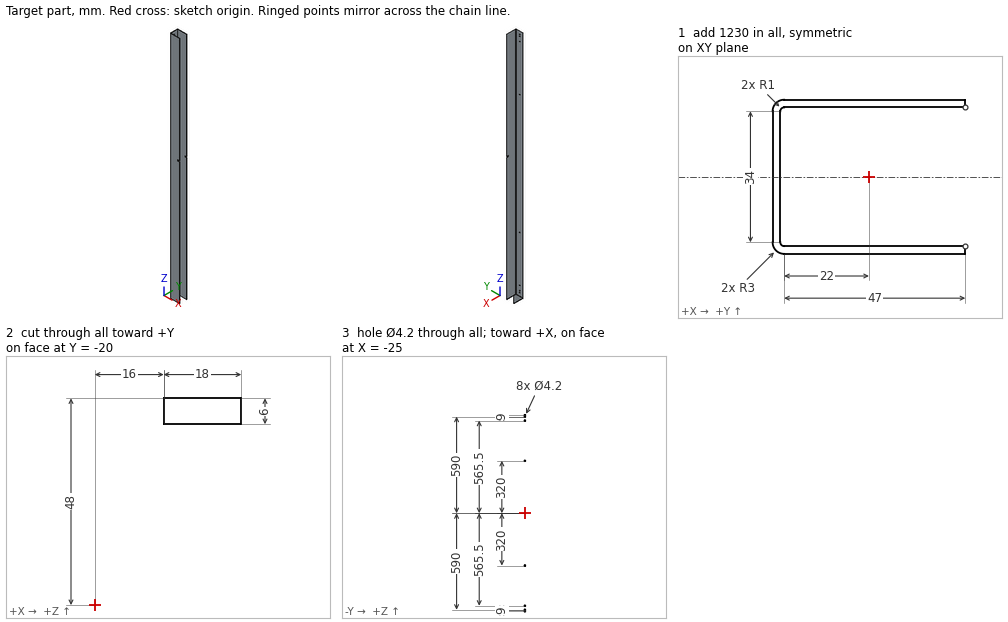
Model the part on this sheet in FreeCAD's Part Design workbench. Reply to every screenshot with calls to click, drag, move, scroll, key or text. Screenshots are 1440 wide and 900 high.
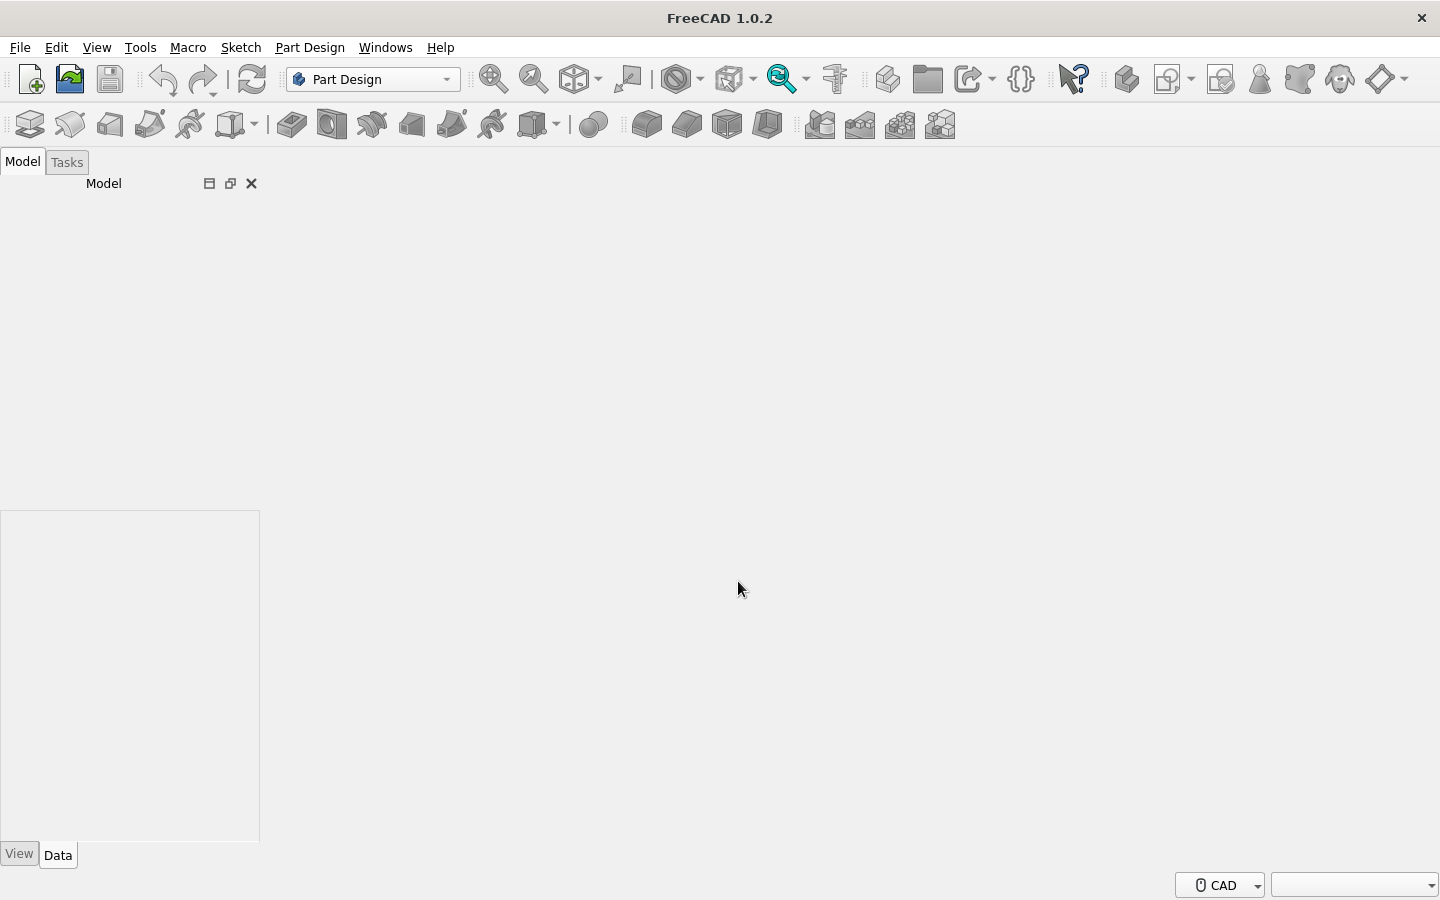
key(ctrl+n)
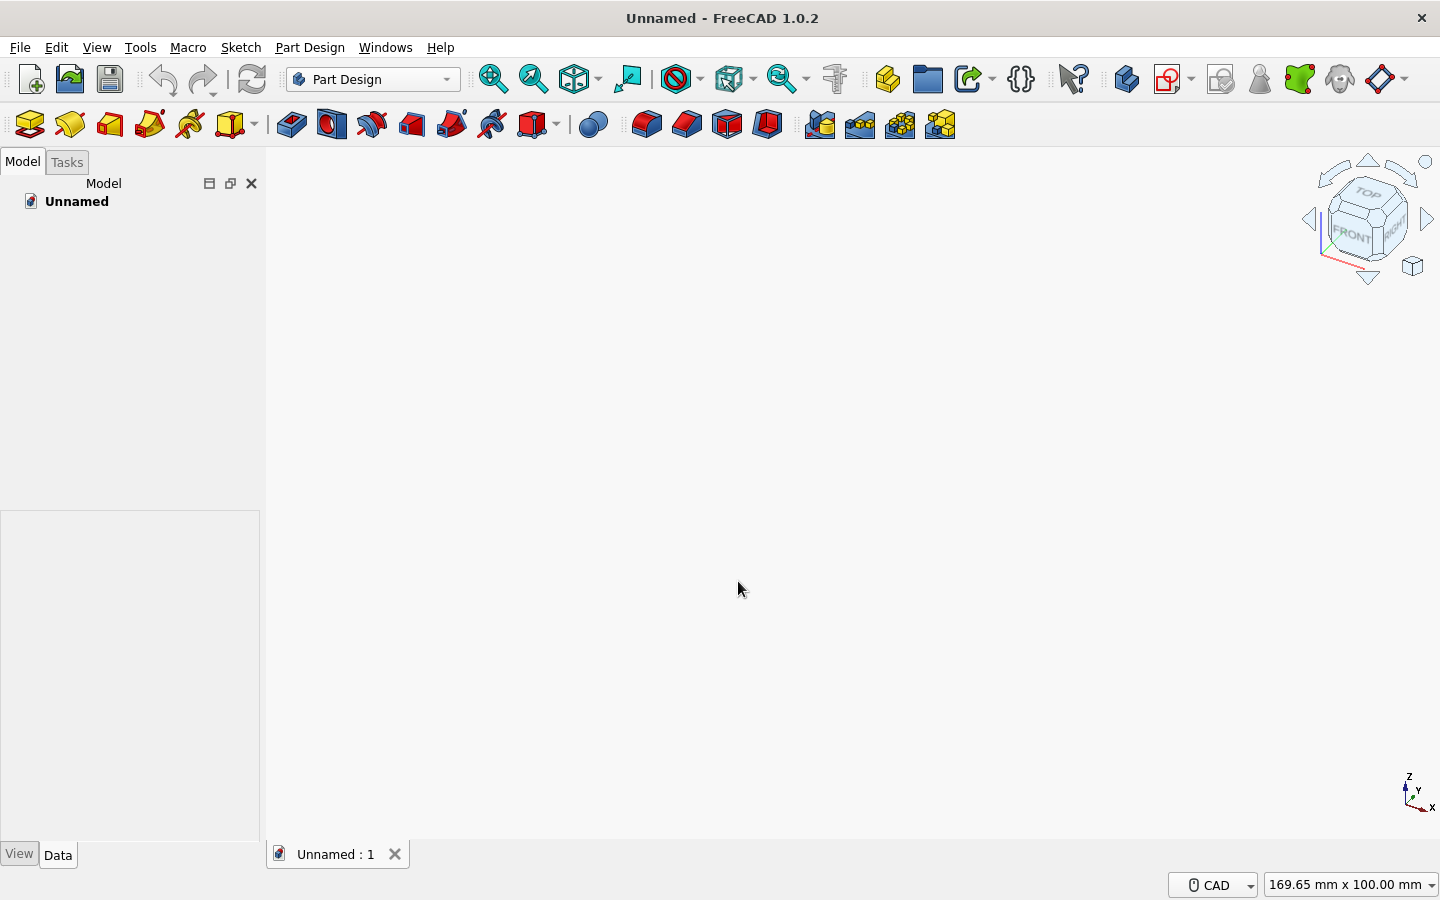
click(1168, 80)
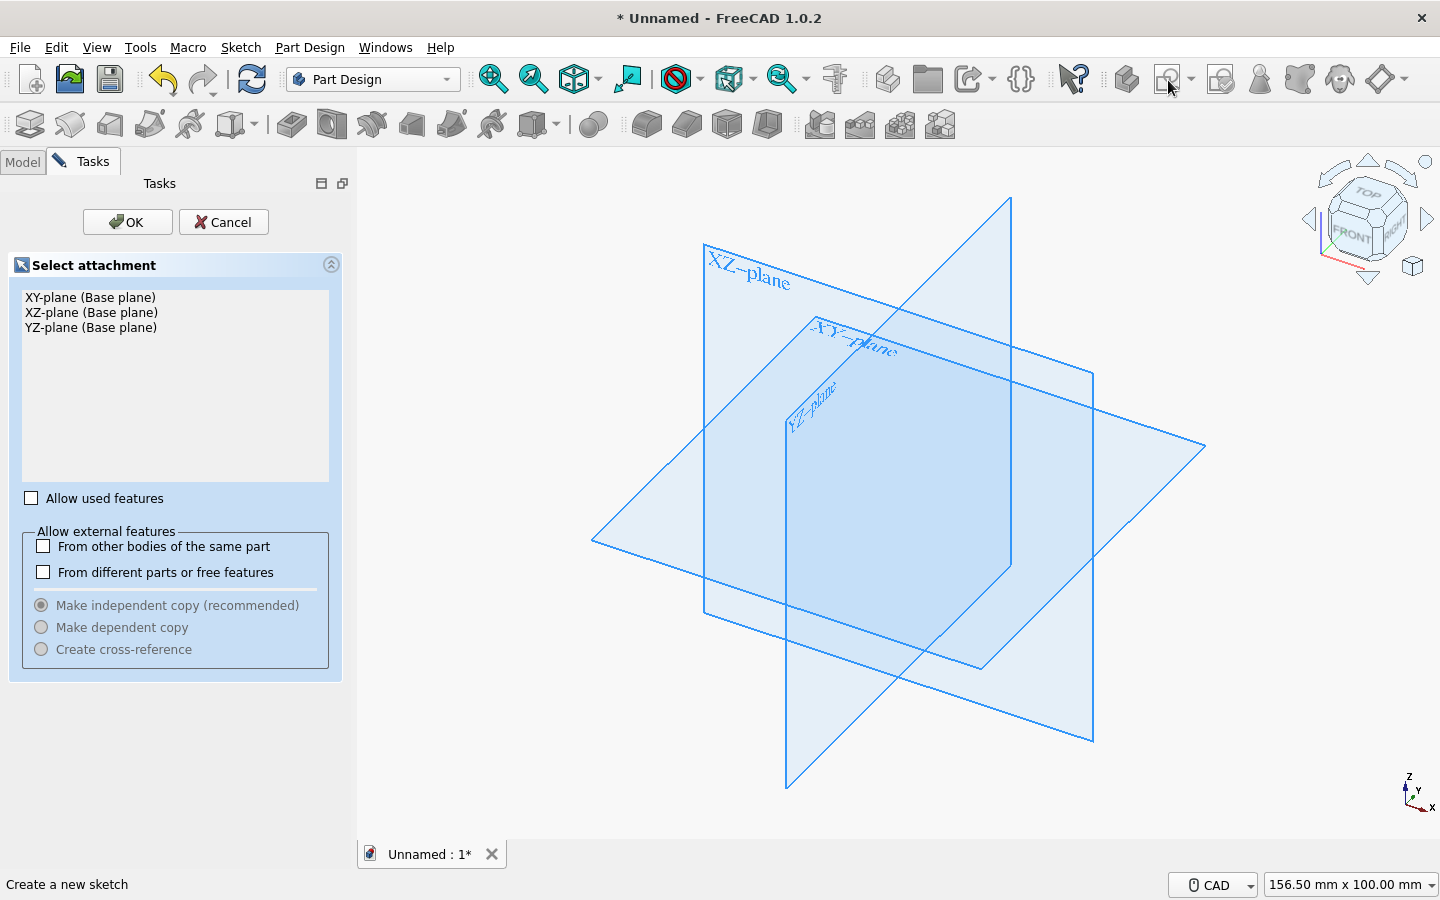
click(82, 298)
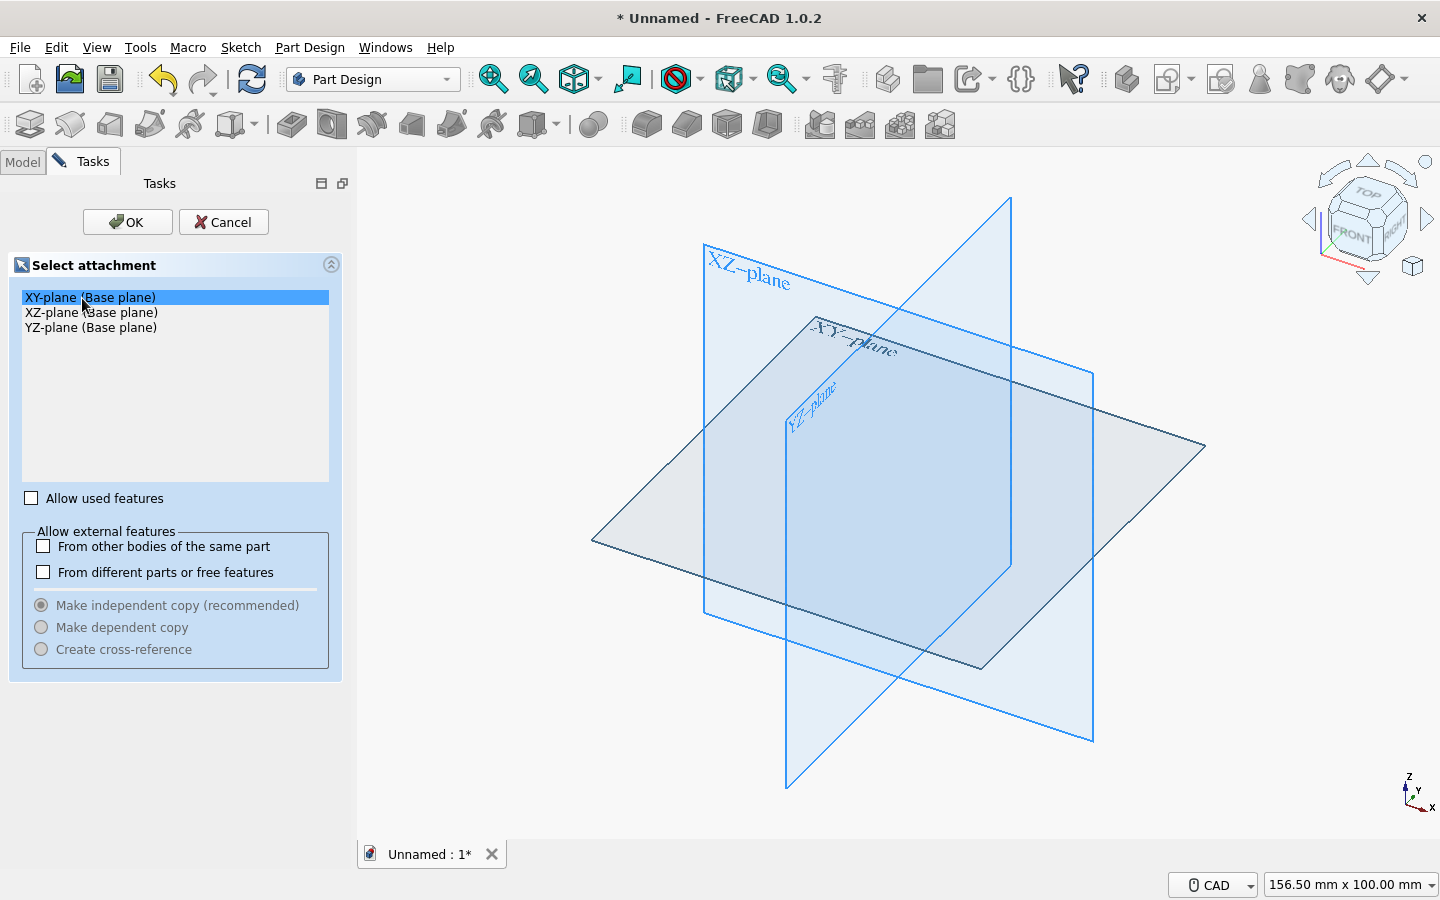
click(128, 222)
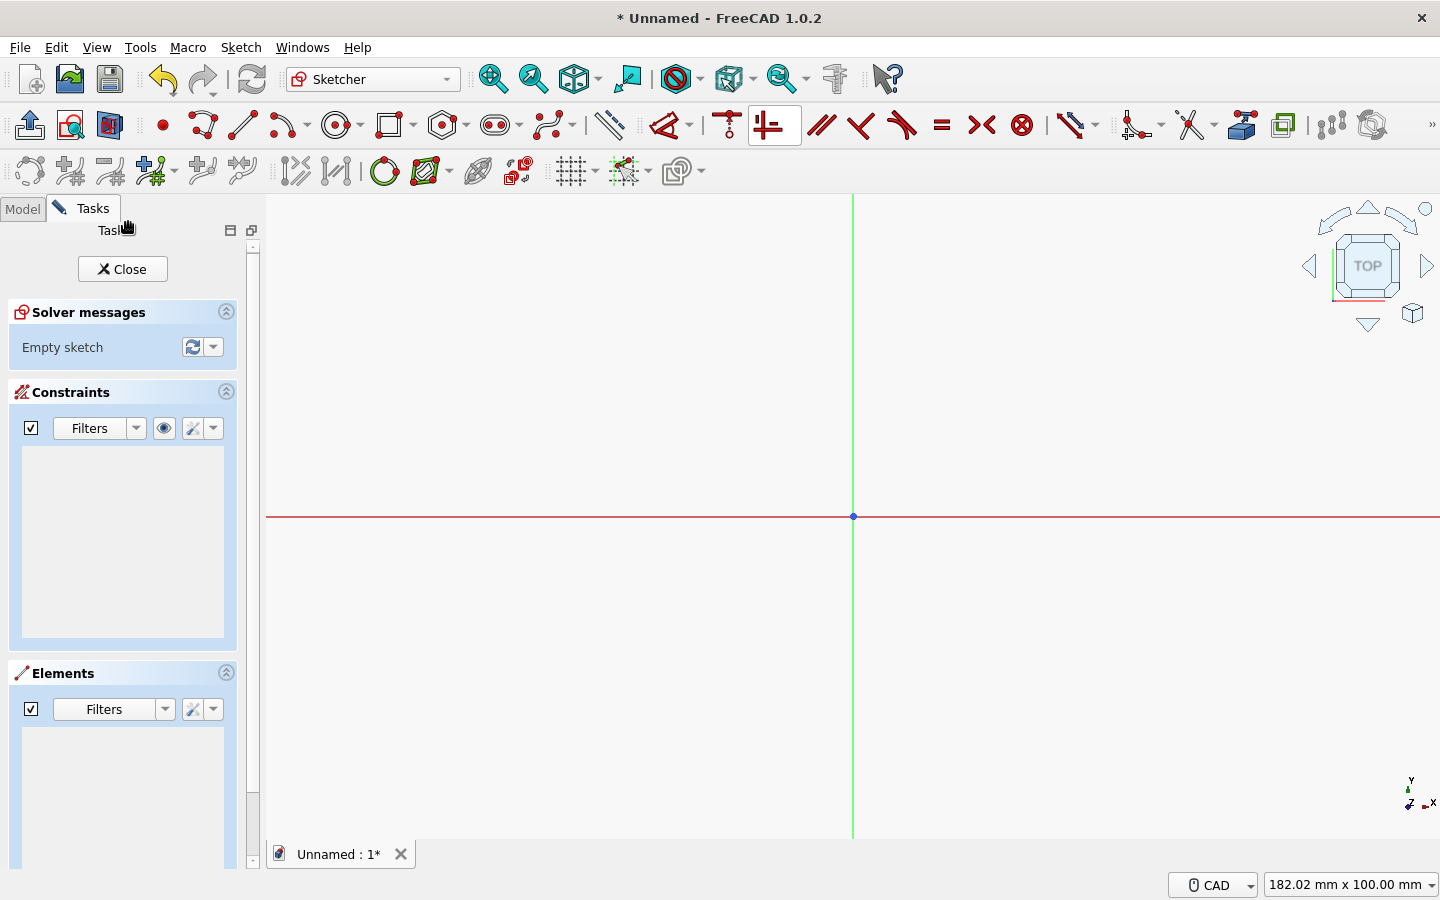
scroll(992, 517, up, 2)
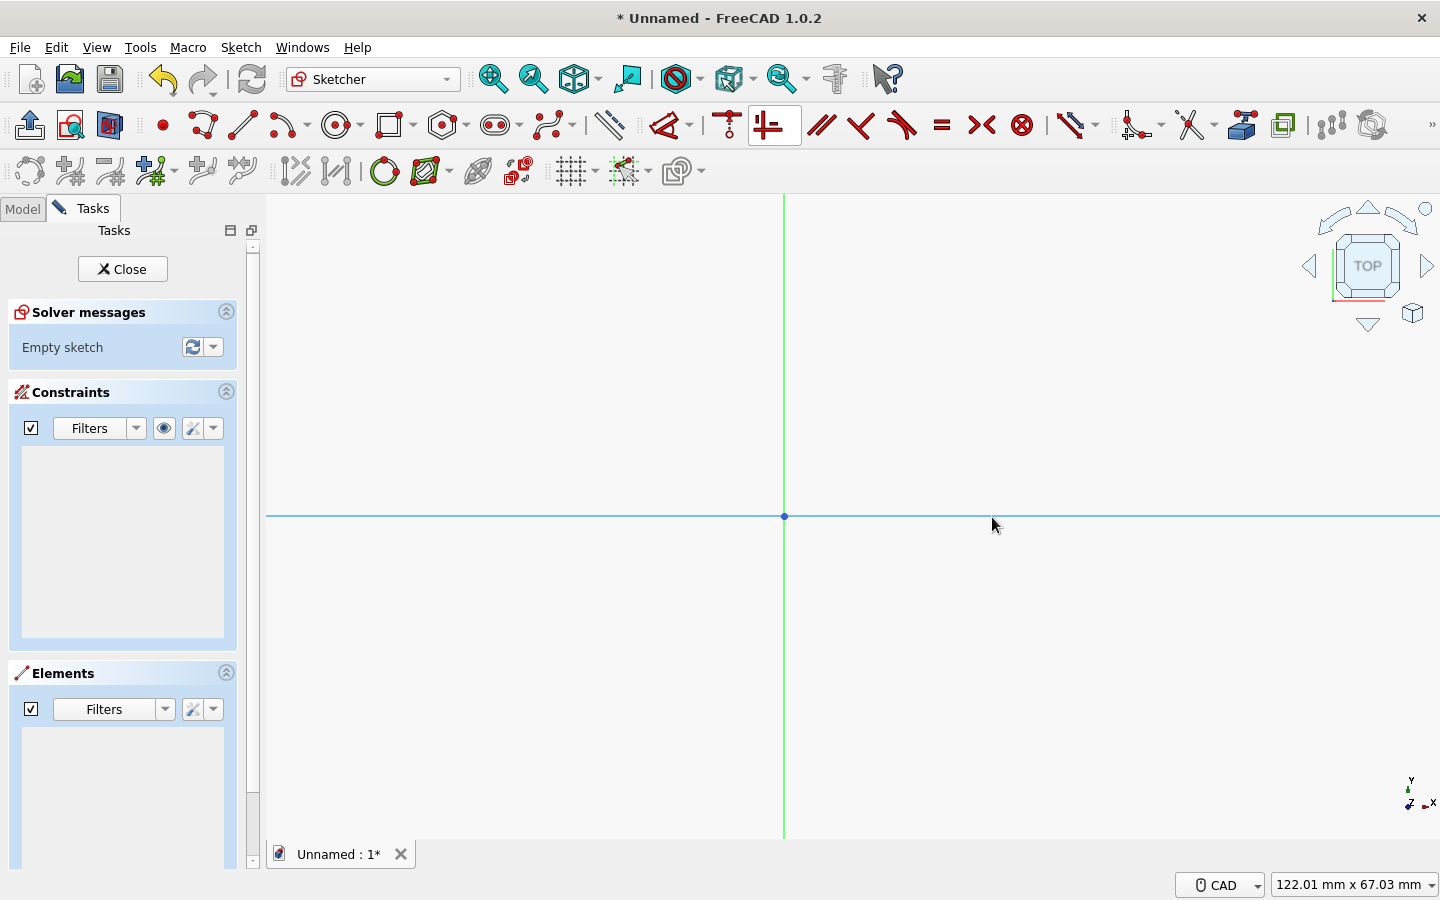
key(g)
key(m)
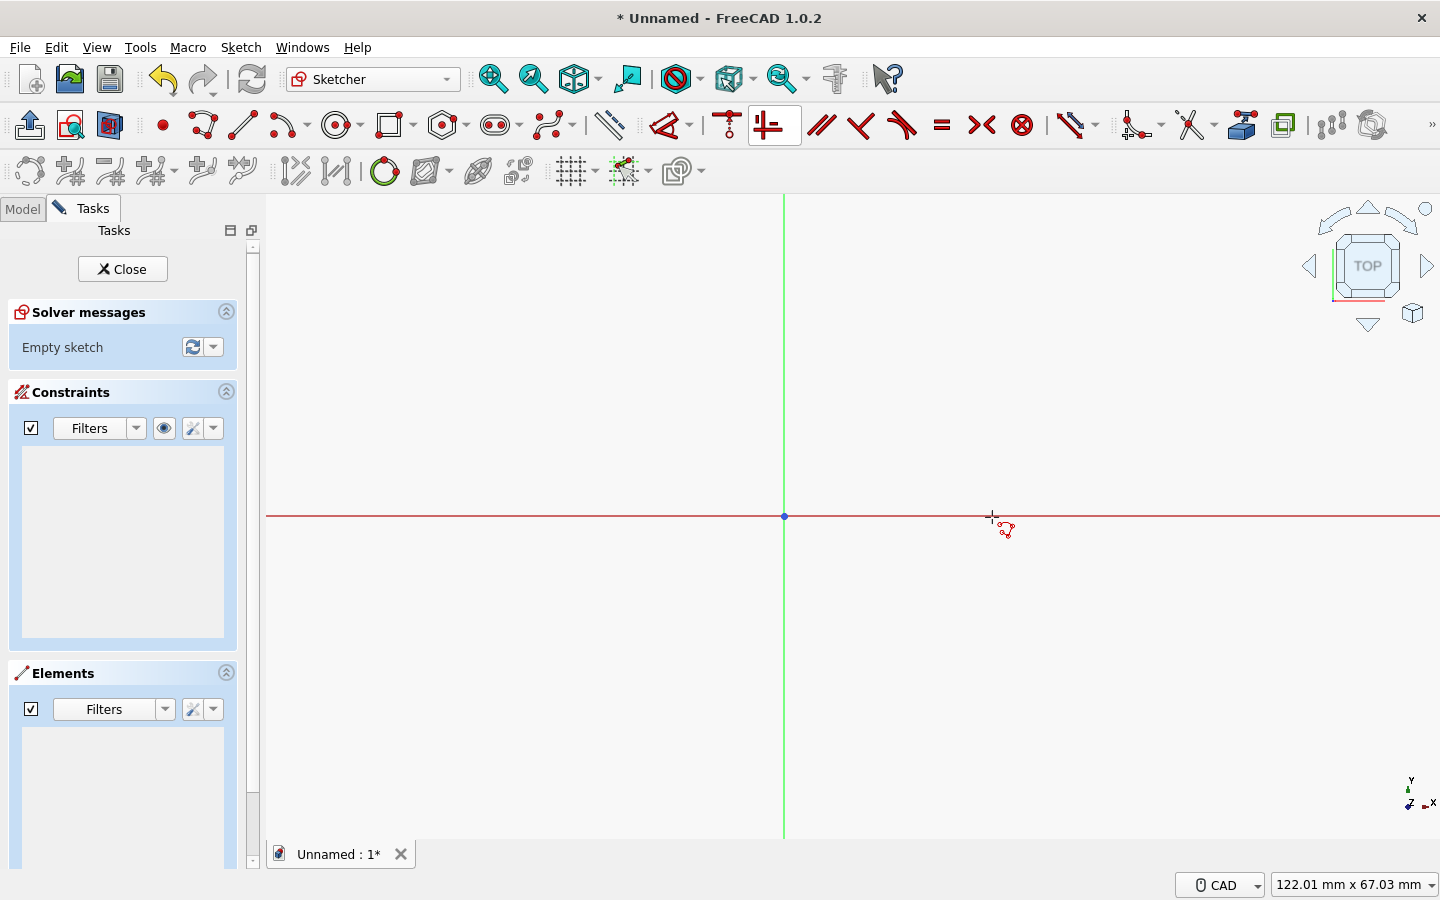
click(573, 708)
click(1025, 708)
click(1025, 689)
click(573, 689)
right_click(573, 689)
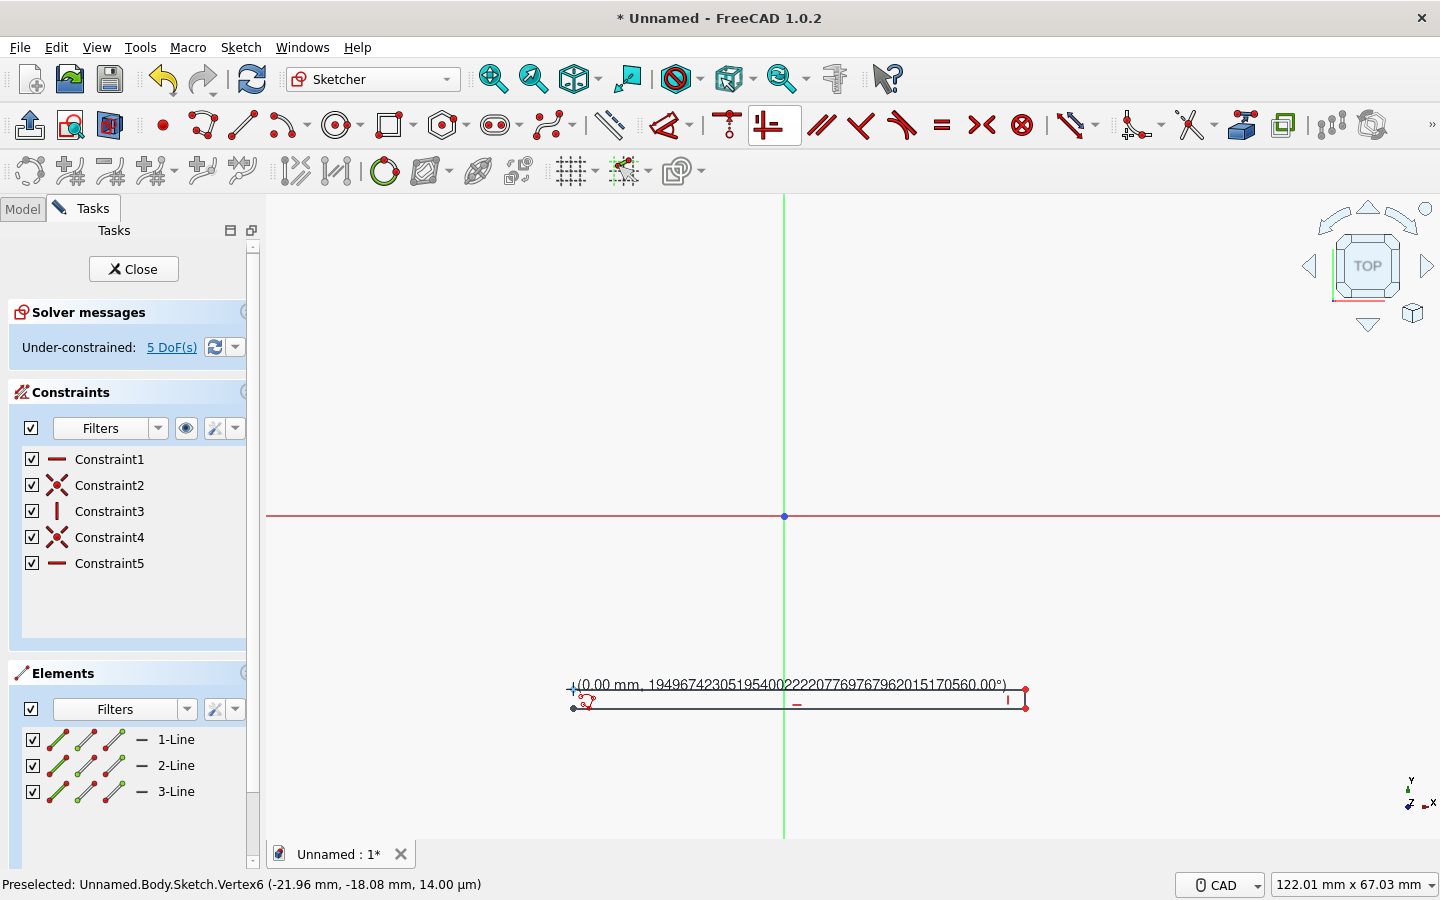
key(g)
key(l)